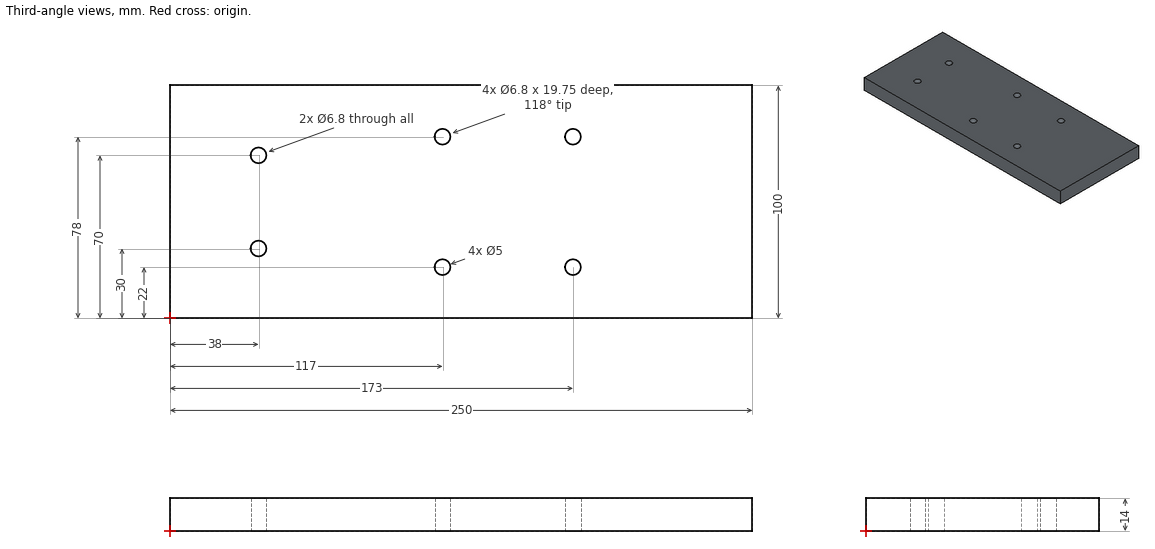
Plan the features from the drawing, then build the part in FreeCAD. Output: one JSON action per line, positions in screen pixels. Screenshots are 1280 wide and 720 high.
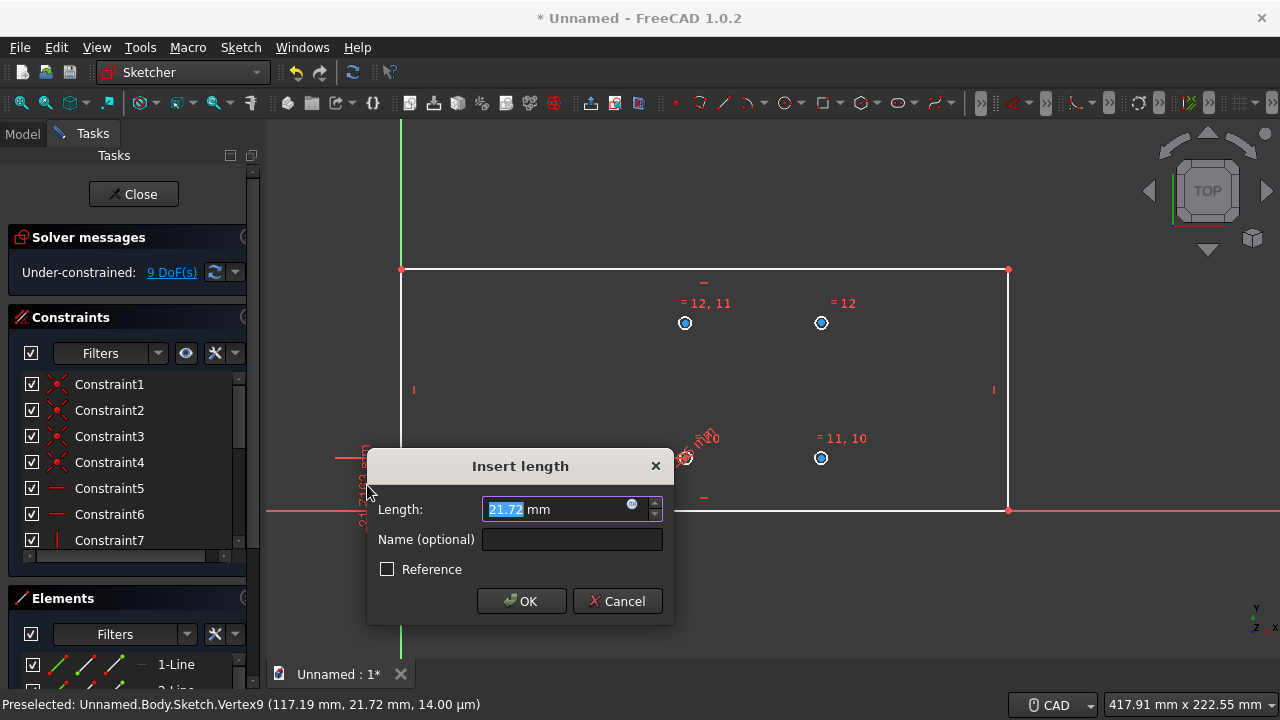
{"action": "type", "text": "22"}
{"action": "key", "text": "Return"}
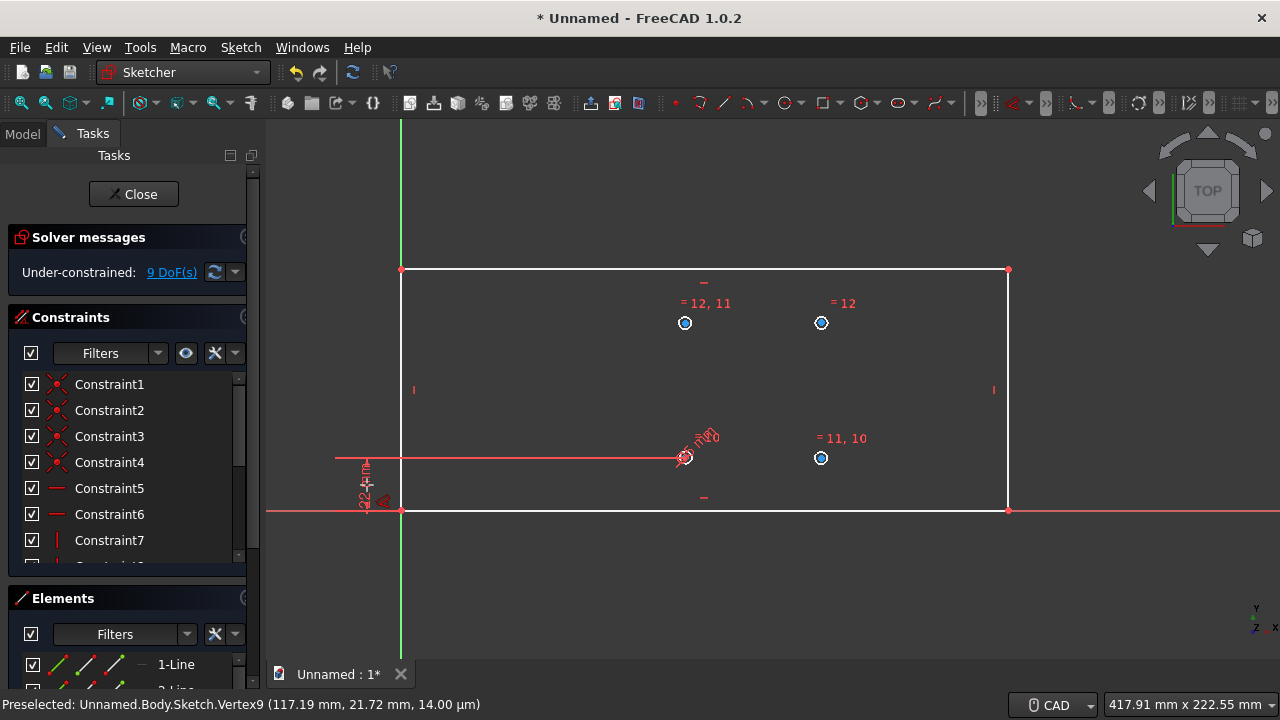
{"action": "left_click", "coordinate": [821, 458]}
{"action": "left_click", "coordinate": [855, 484]}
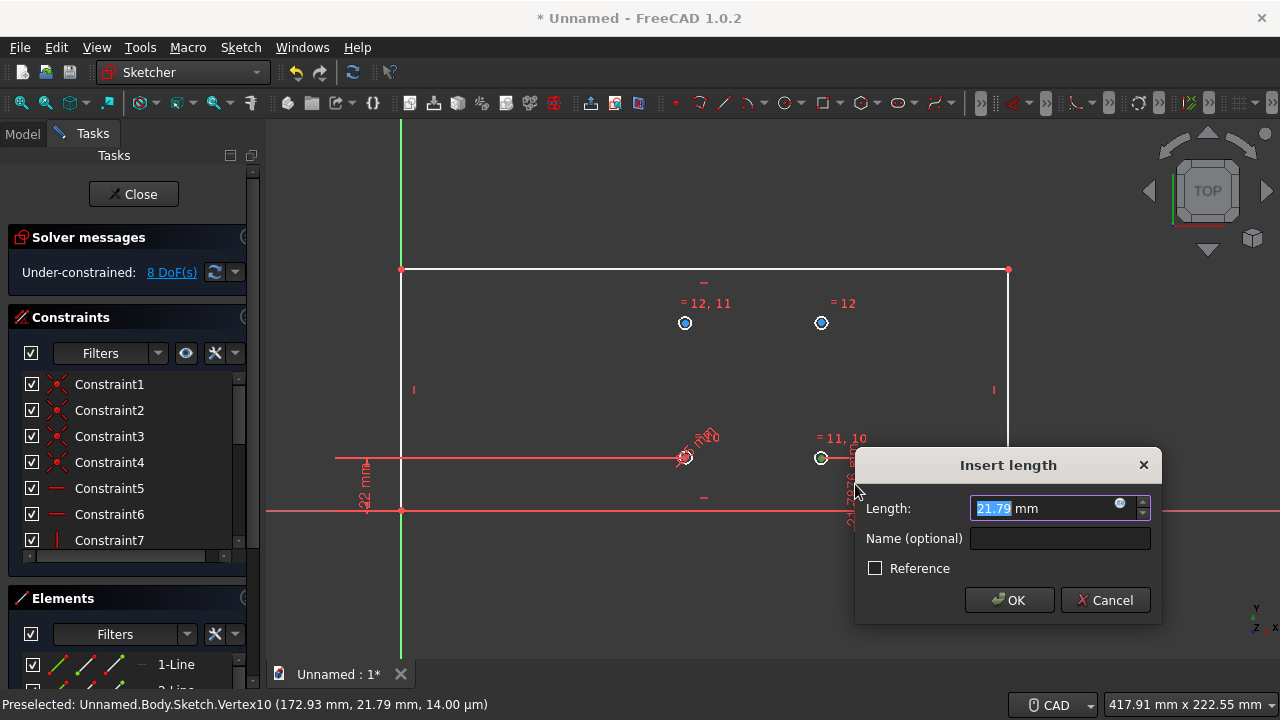
{"action": "type", "text": "22"}
{"action": "key", "text": "Return"}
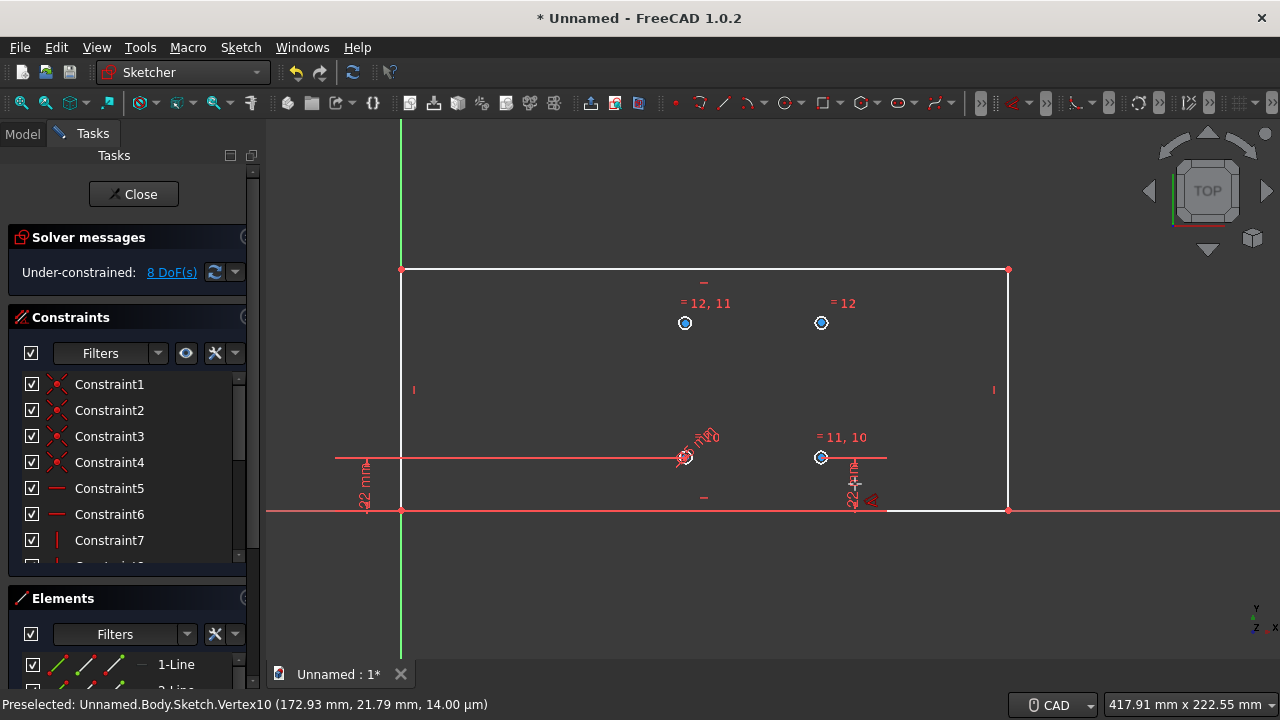
{"action": "left_click", "coordinate": [685, 323]}
{"action": "left_click", "coordinate": [367, 417]}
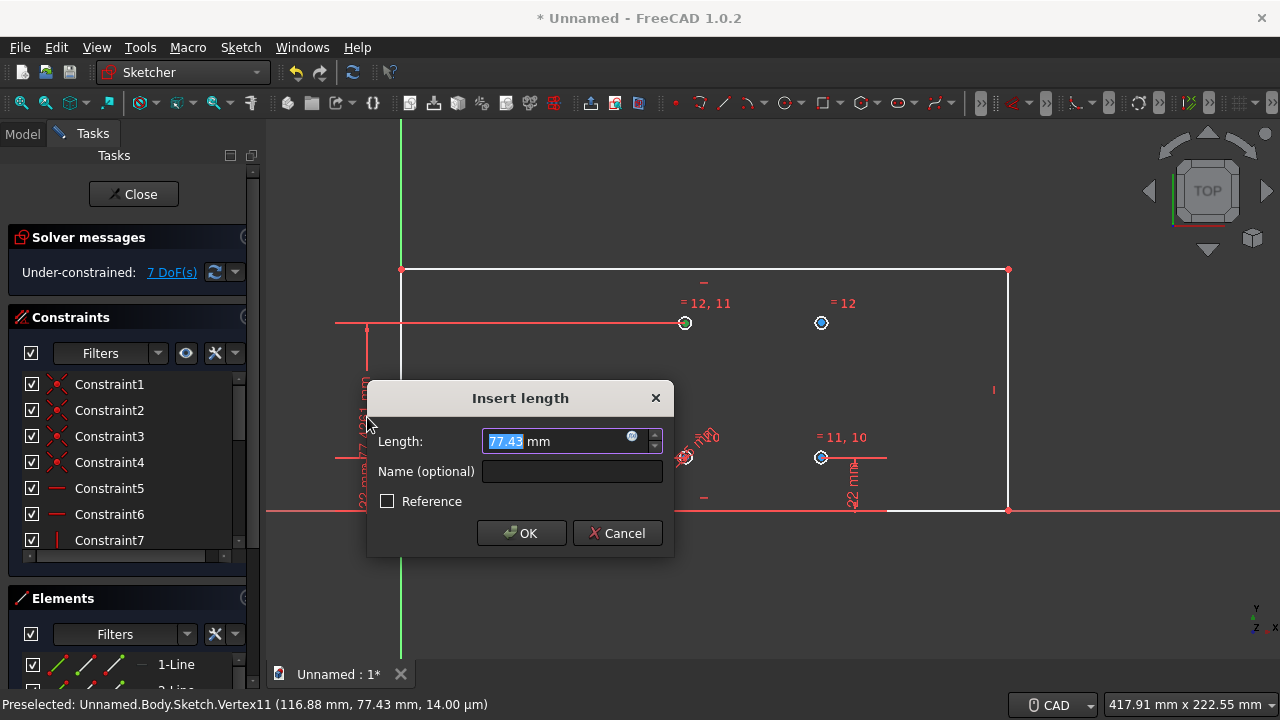
{"action": "type", "text": "78"}
{"action": "key", "text": "Return"}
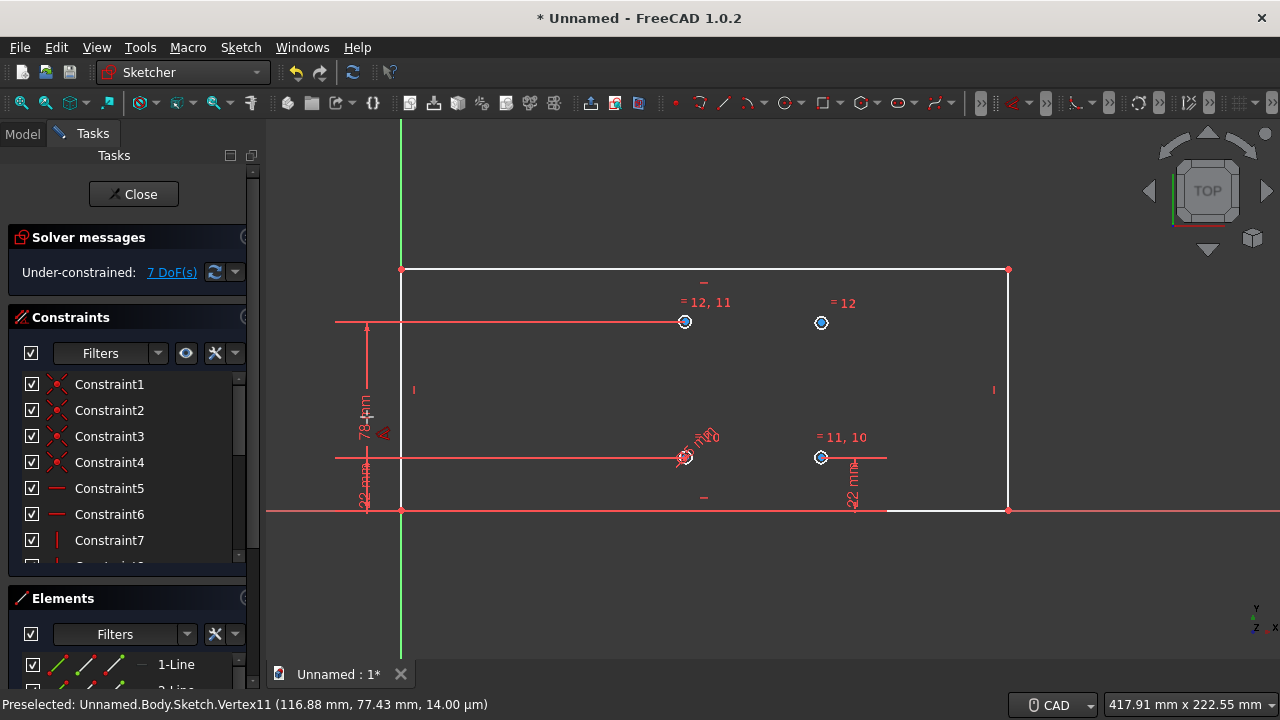
{"action": "left_click", "coordinate": [822, 323]}
{"action": "left_click", "coordinate": [367, 374]}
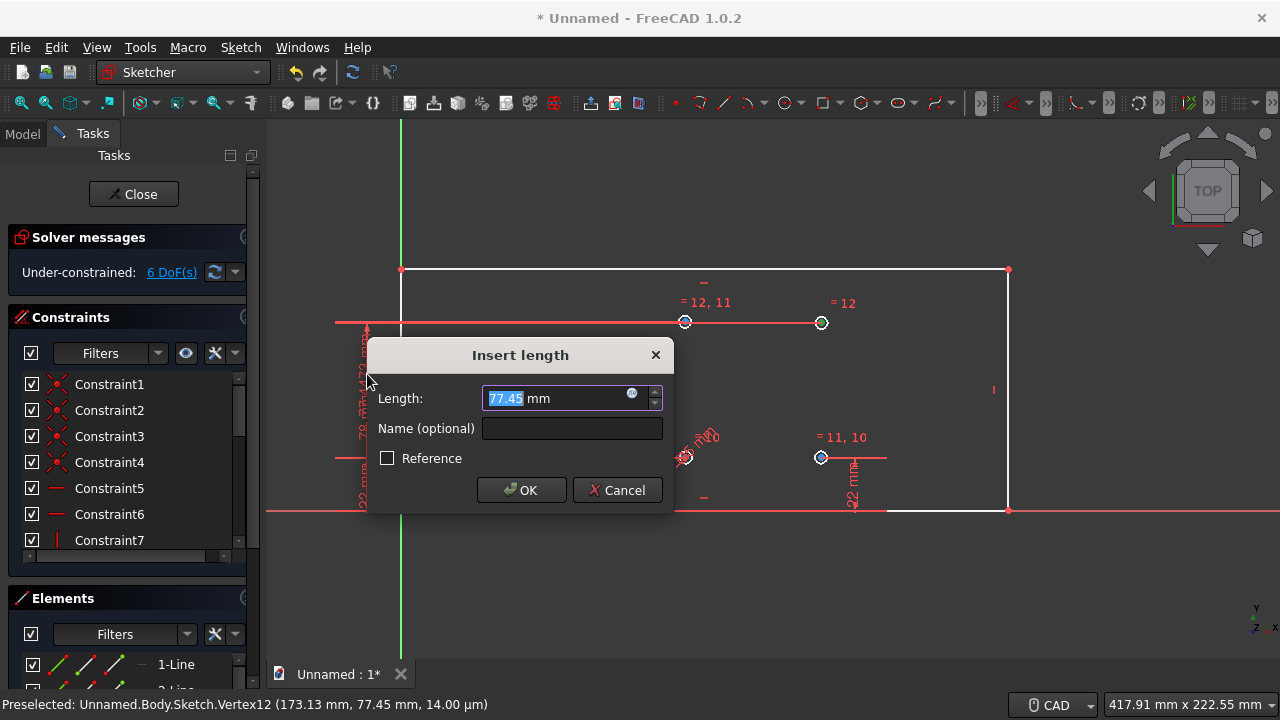
{"action": "type", "text": "78"}
{"action": "key", "text": "Return"}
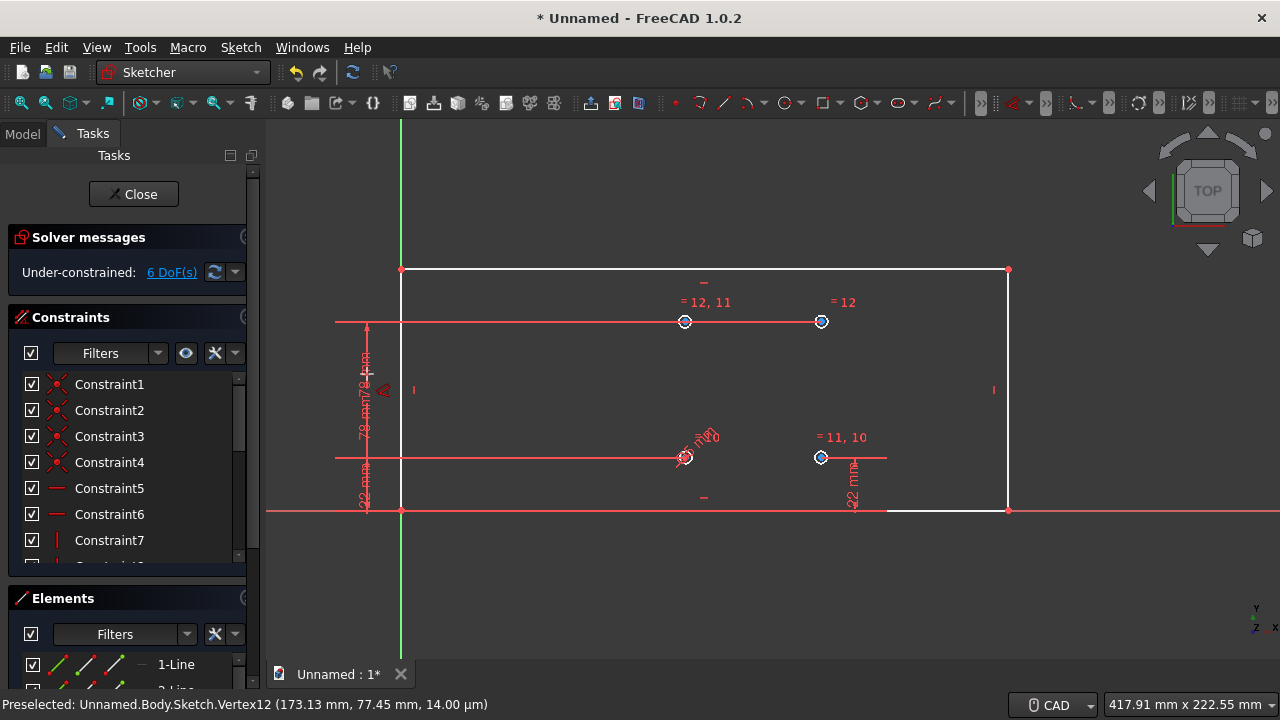
{"action": "left_click", "coordinate": [583, 511]}
{"action": "left_click", "coordinate": [705, 545]}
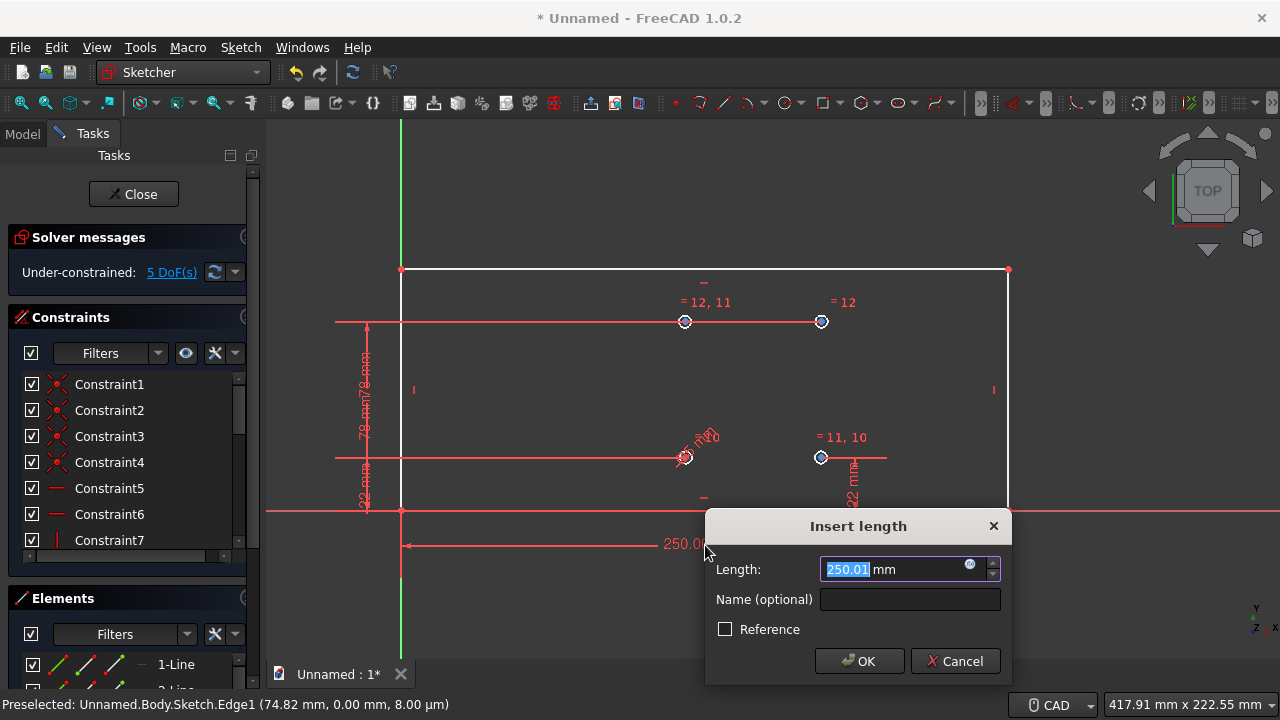
{"action": "type", "text": "250"}
{"action": "key", "text": "Return"}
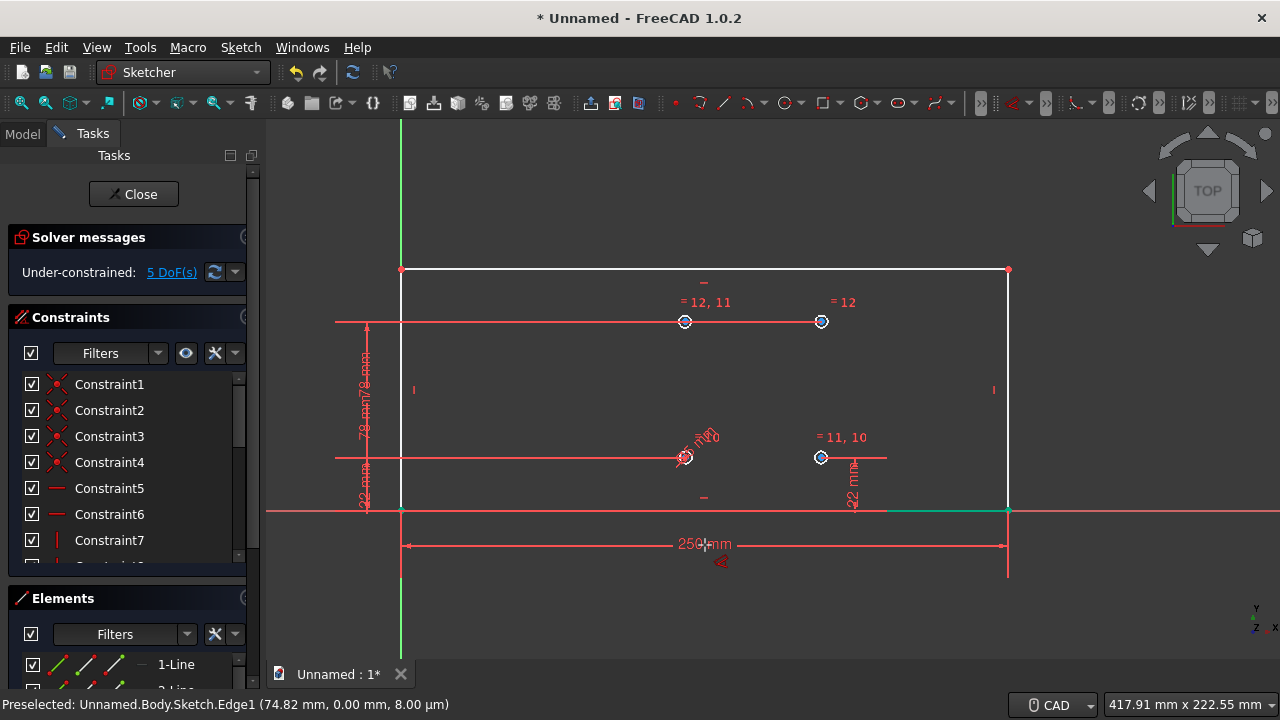
{"action": "left_click", "coordinate": [1008, 438]}
{"action": "left_click", "coordinate": [1042, 390]}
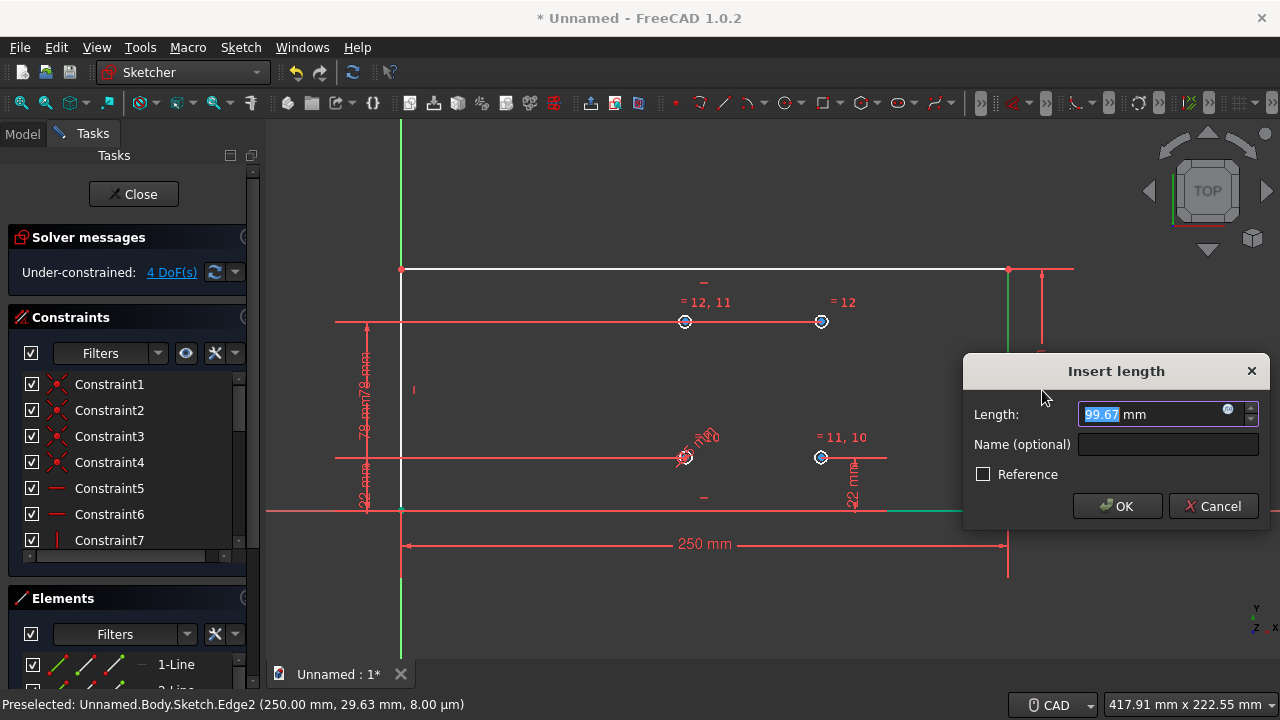
{"action": "type", "text": "100"}
{"action": "key", "text": "Return"}